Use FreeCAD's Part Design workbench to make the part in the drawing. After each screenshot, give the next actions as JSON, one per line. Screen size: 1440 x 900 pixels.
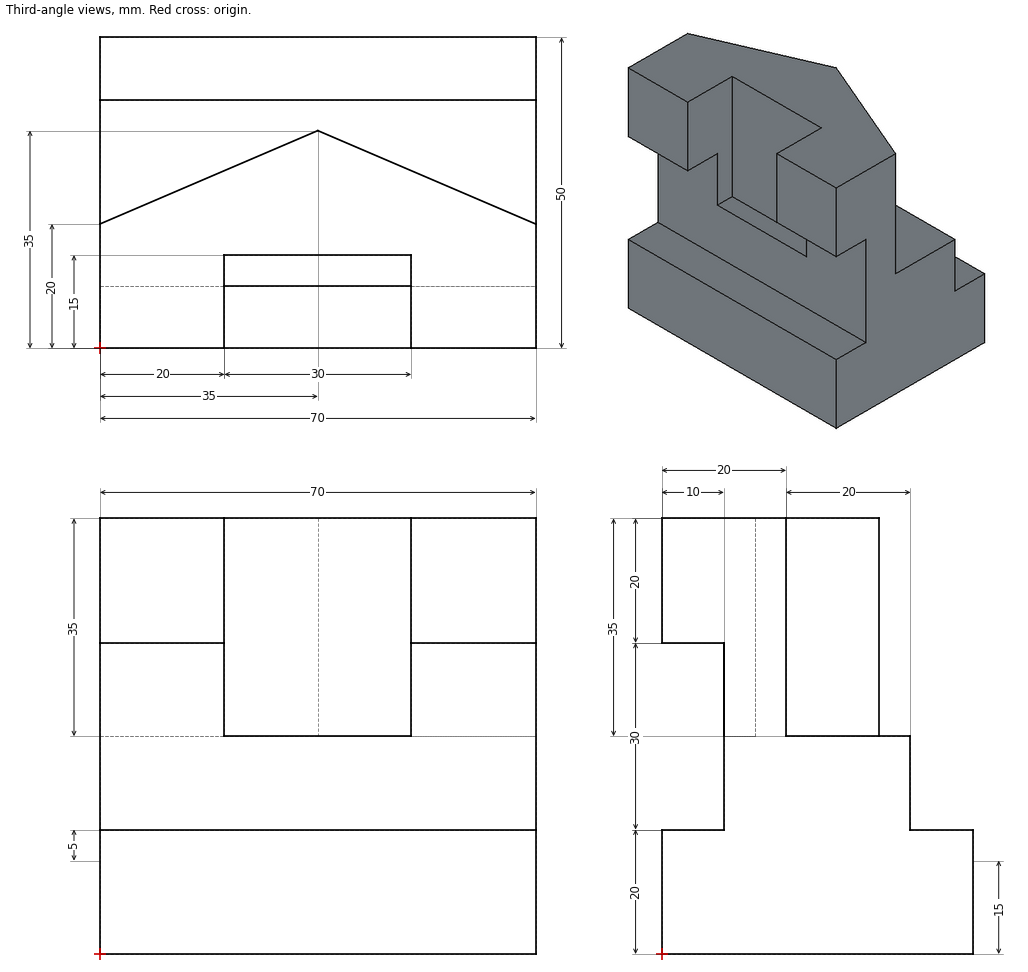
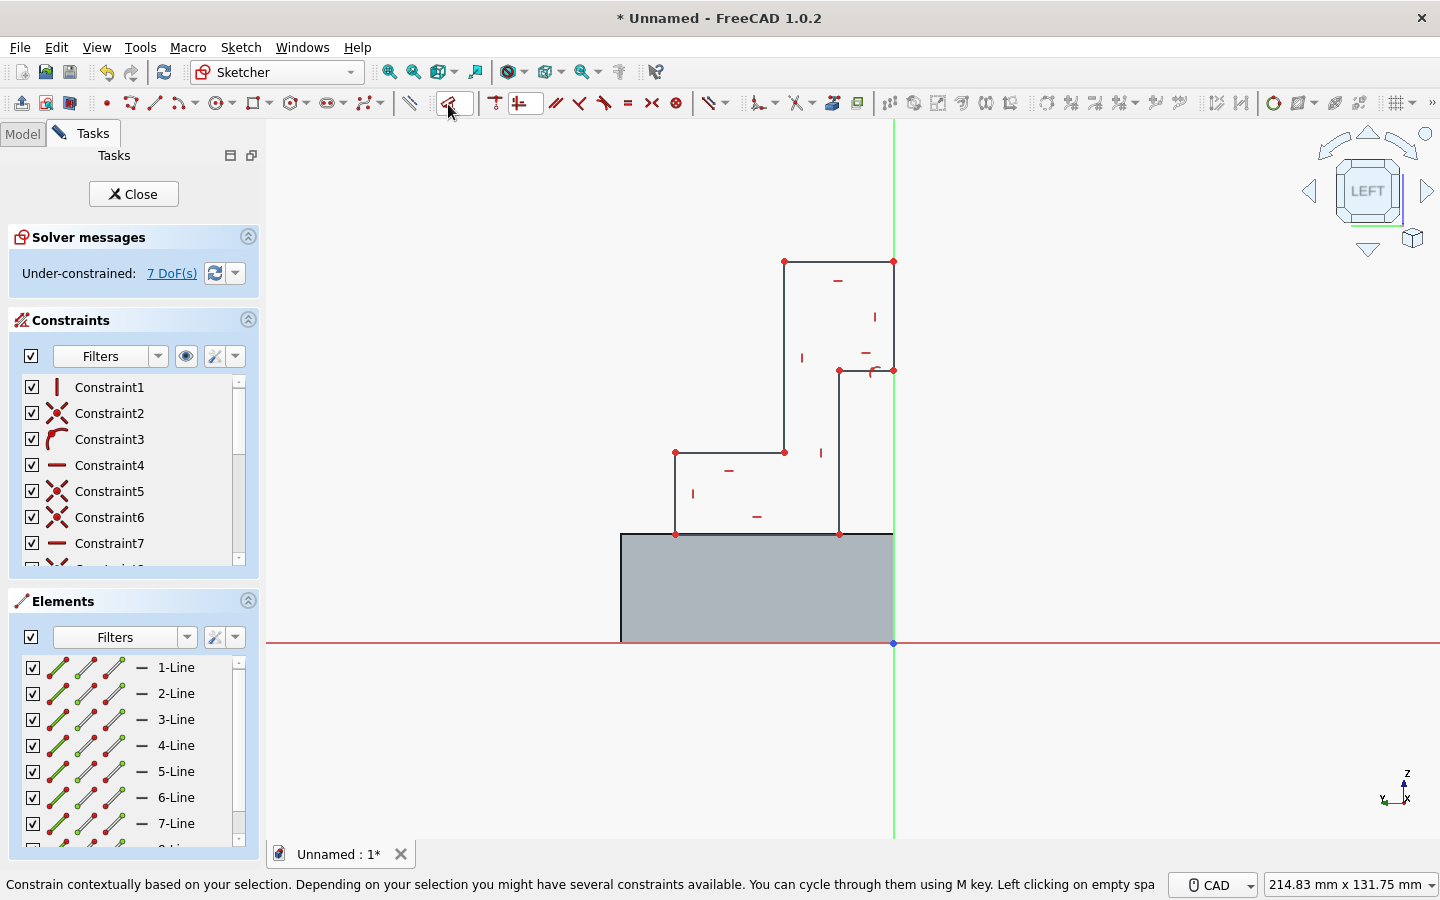
{"action": "left_click", "coordinate": [839, 486]}
{"action": "left_click", "coordinate": [873, 453]}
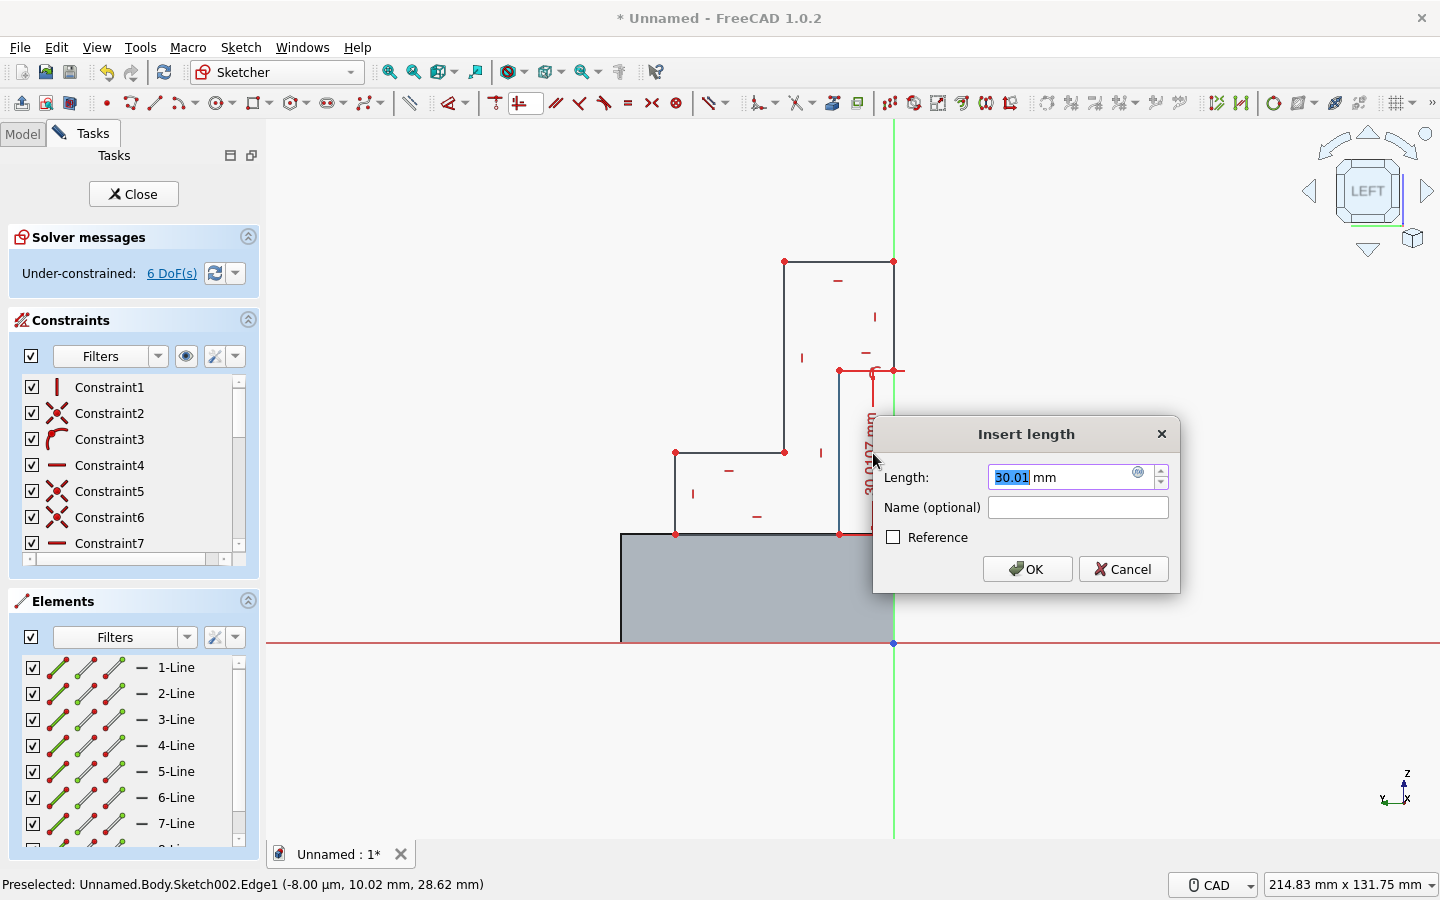
{"action": "type", "text": "30"}
{"action": "key", "text": "Return"}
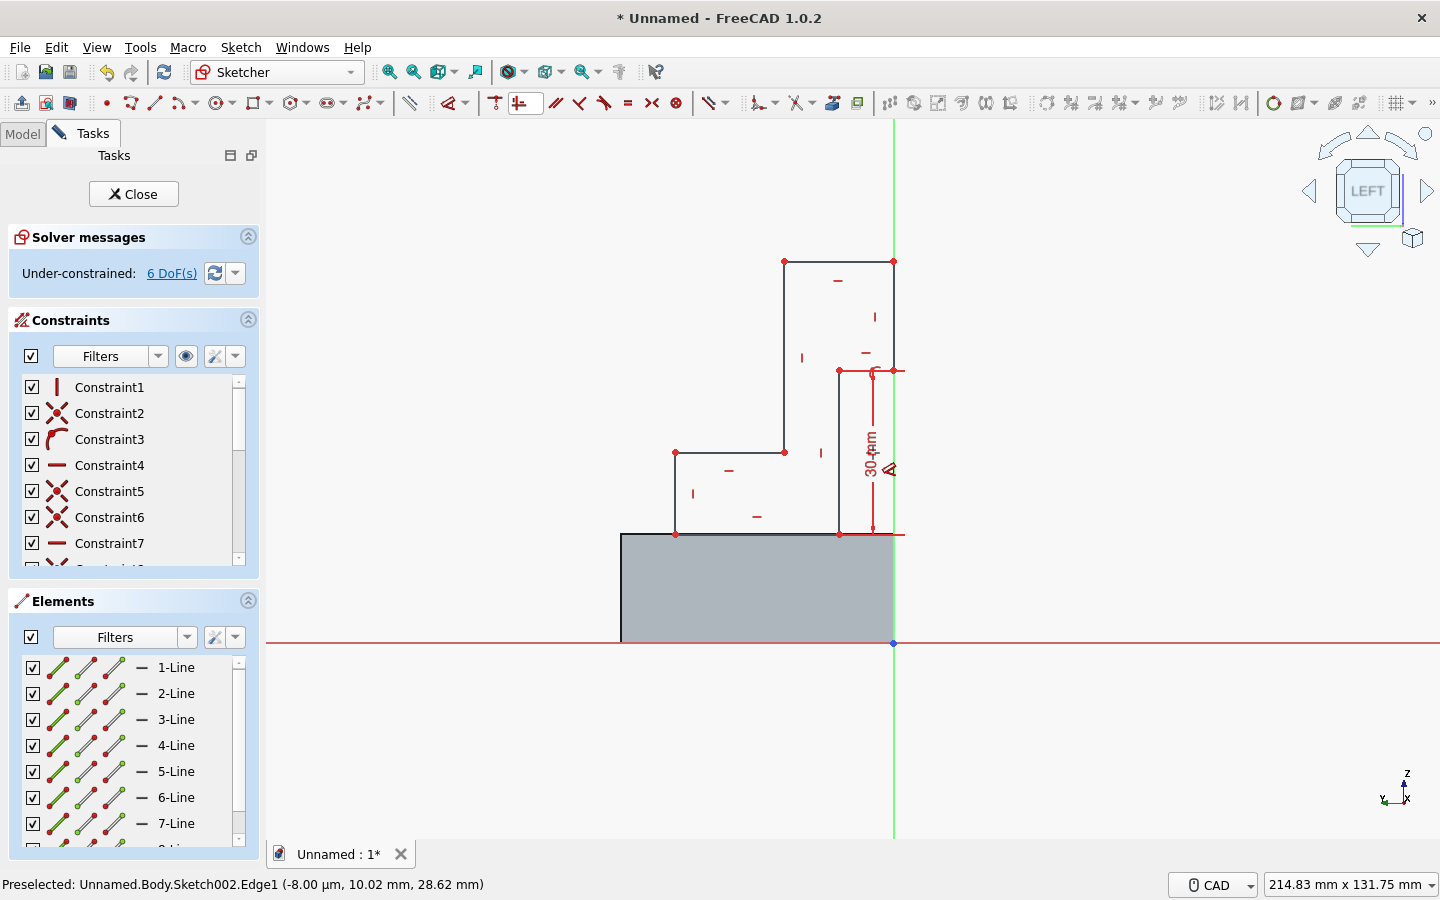
{"action": "left_click", "coordinate": [855, 371]}
{"action": "left_click", "coordinate": [866, 337]}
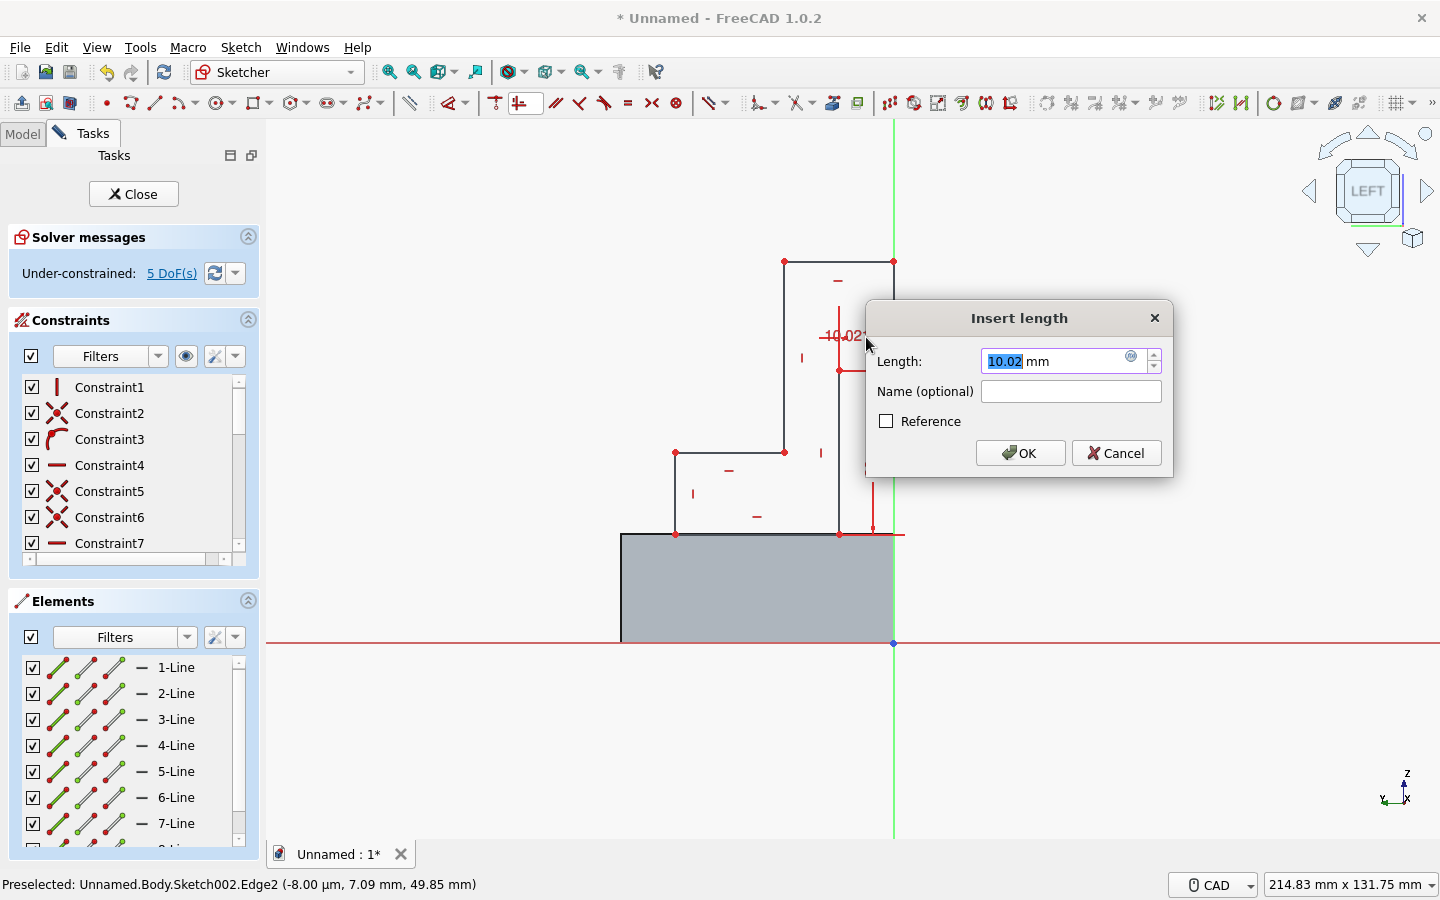
{"action": "type", "text": "10"}
{"action": "key", "text": "Return"}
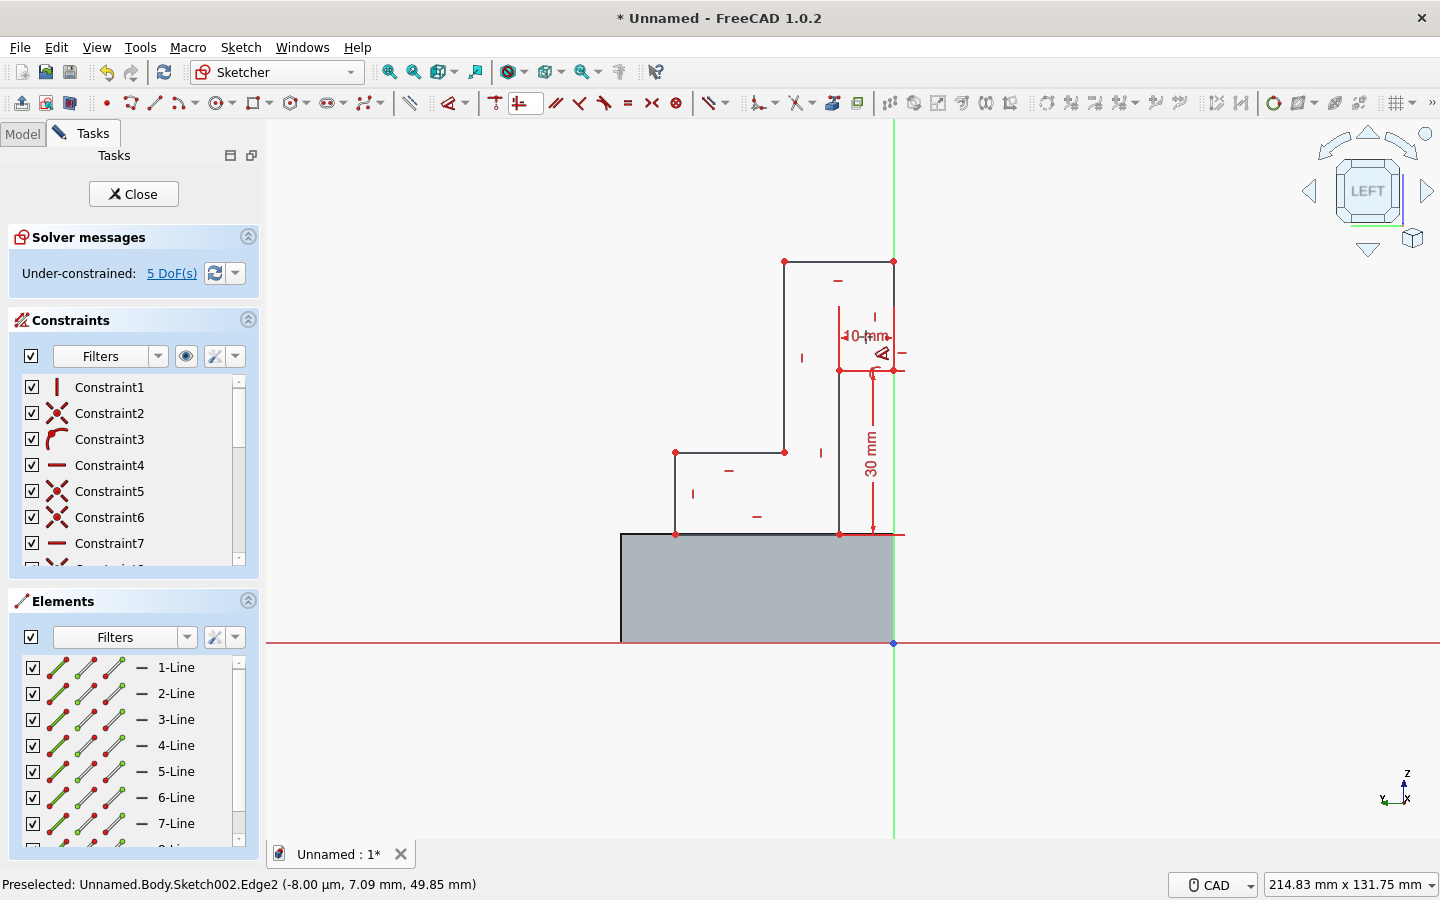
{"action": "left_click", "coordinate": [894, 338]}
{"action": "left_click", "coordinate": [928, 317]}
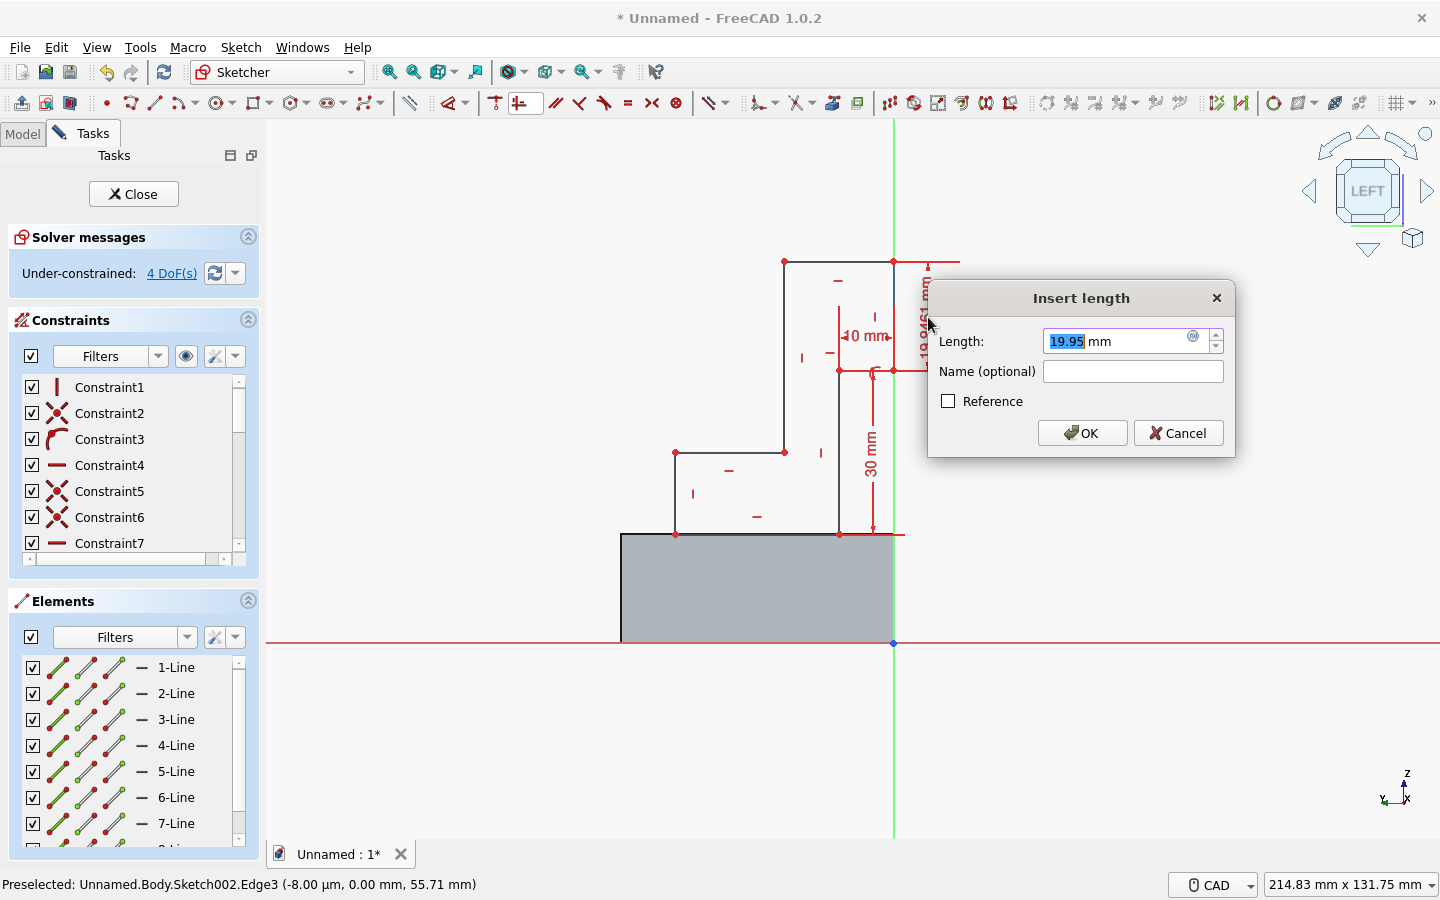
{"action": "type", "text": "20"}
{"action": "key", "text": "Return"}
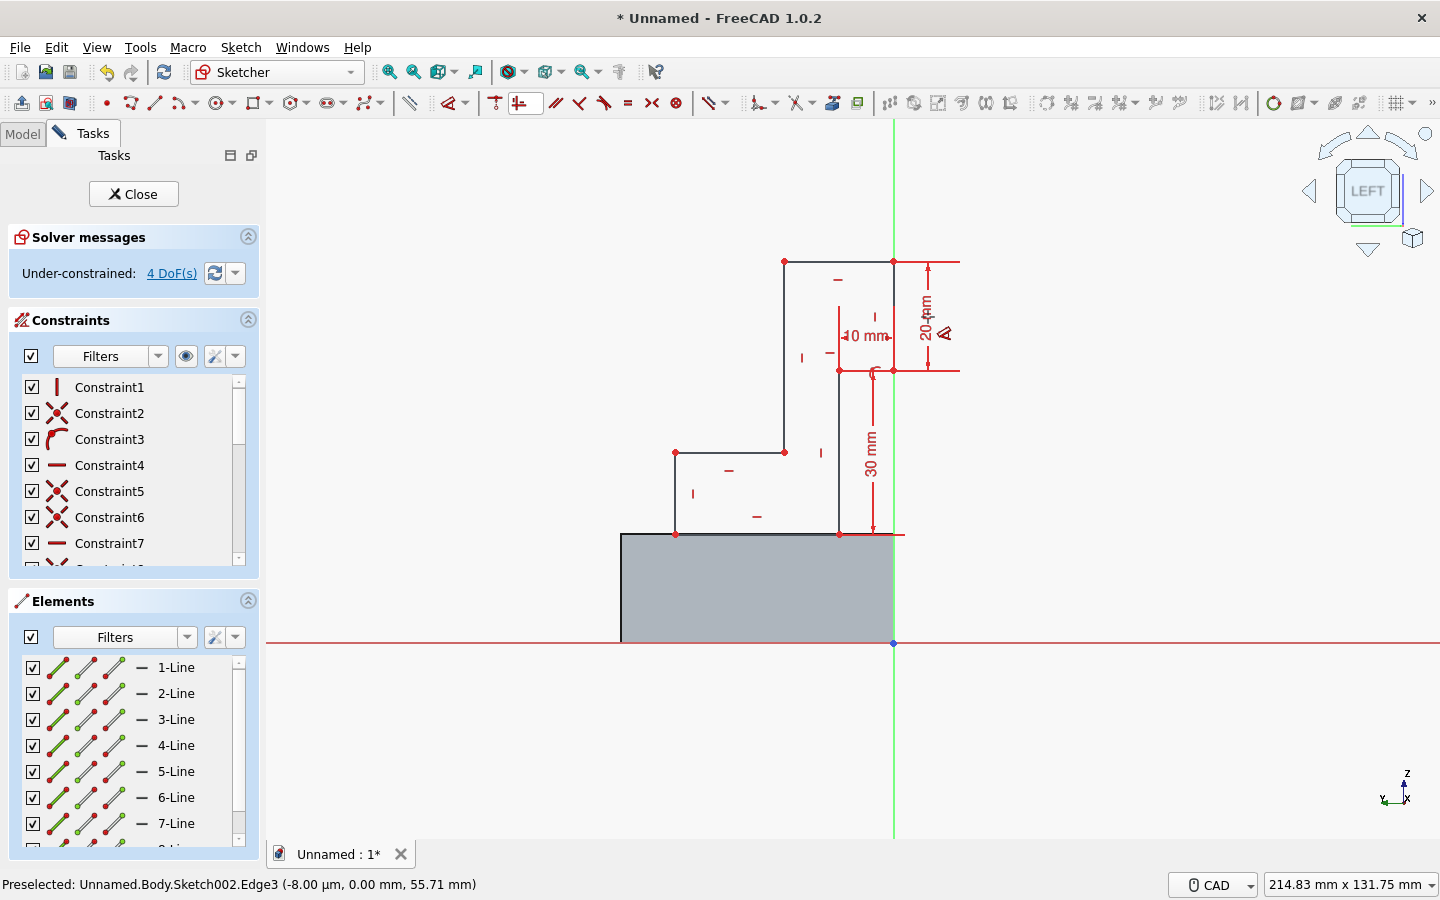
{"action": "left_click", "coordinate": [861, 262]}
{"action": "left_click", "coordinate": [839, 228]}